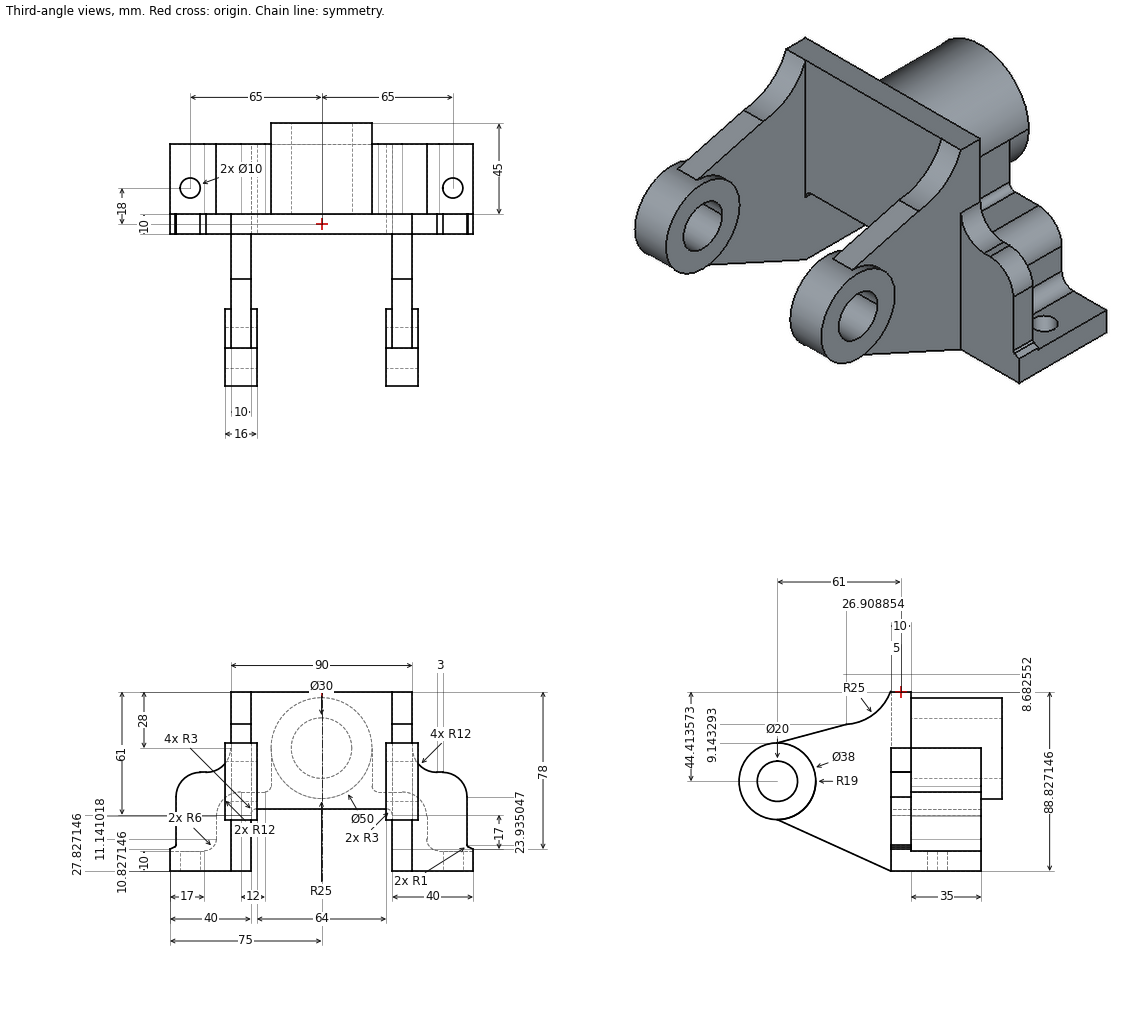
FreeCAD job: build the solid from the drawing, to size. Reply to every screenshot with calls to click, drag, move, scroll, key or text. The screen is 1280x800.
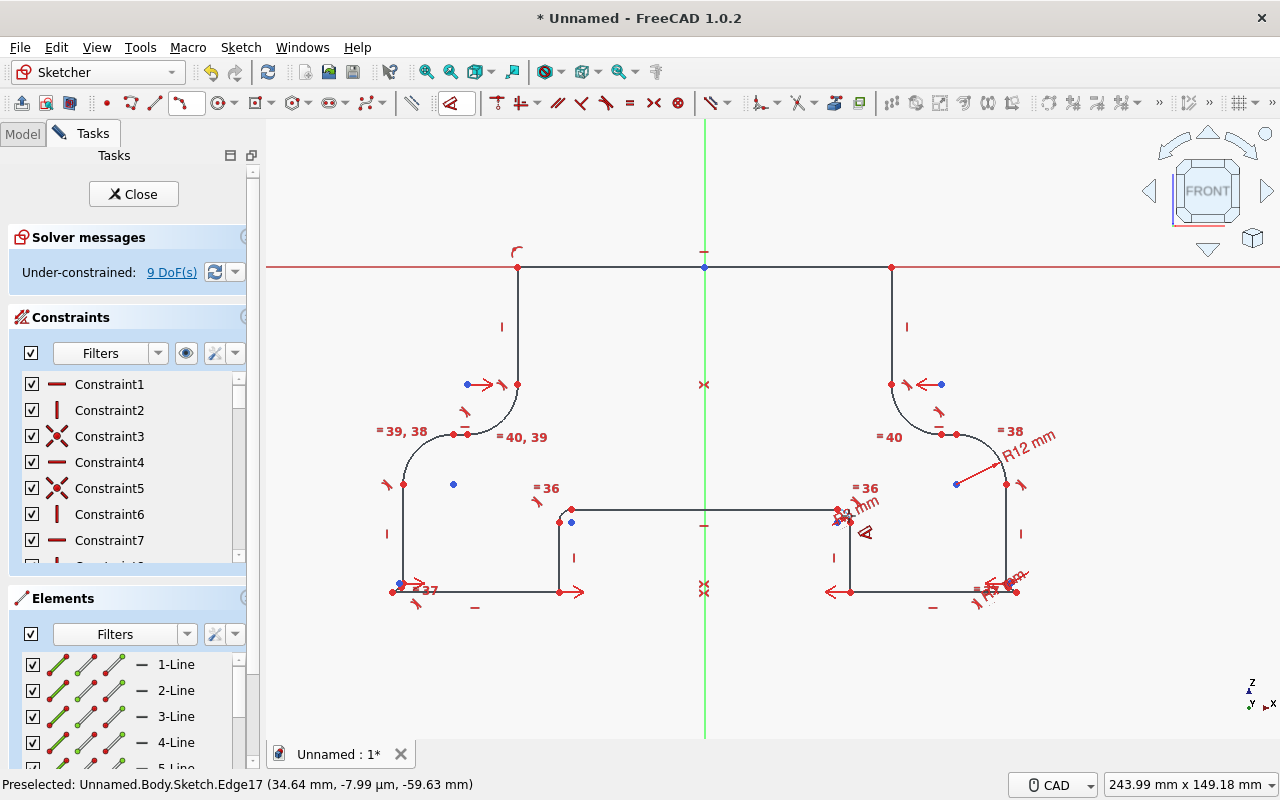
scroll(946, 435, up, 6)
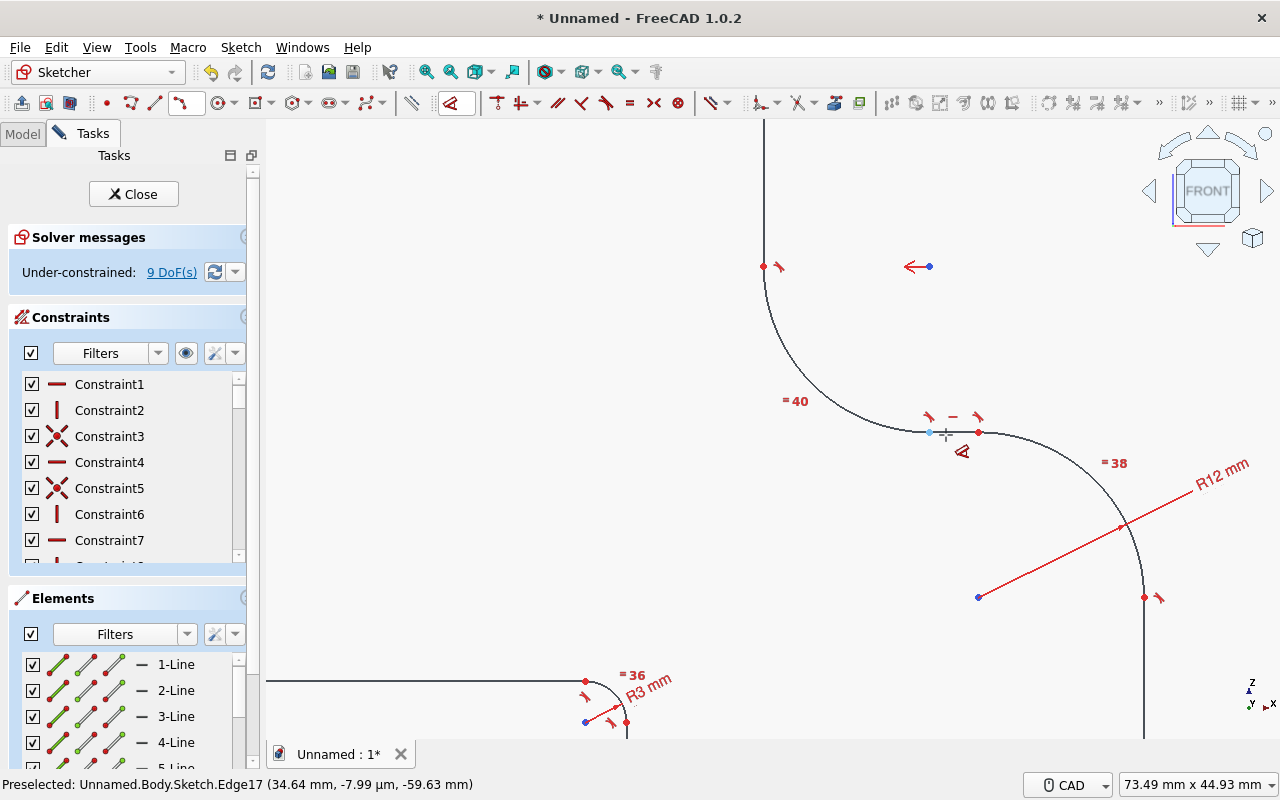
click(944, 432)
click(954, 466)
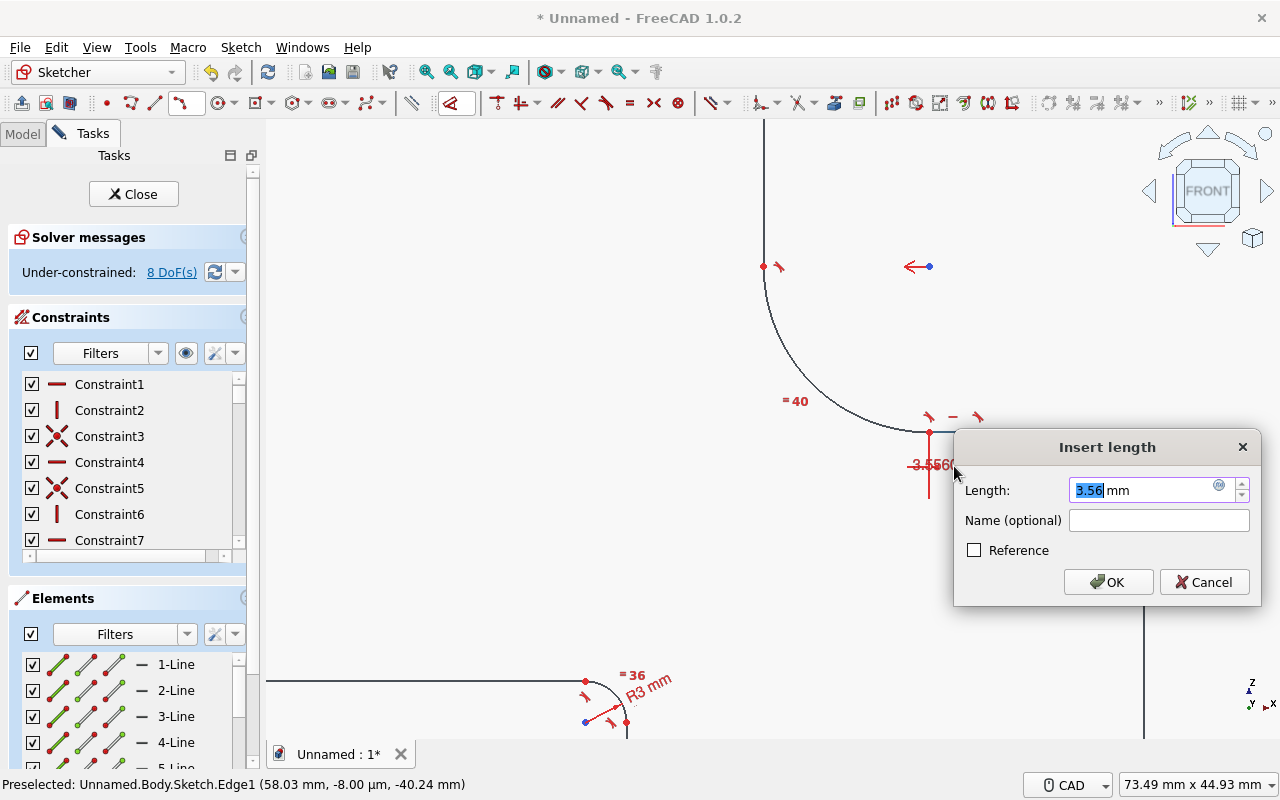
text(3)
key(Return)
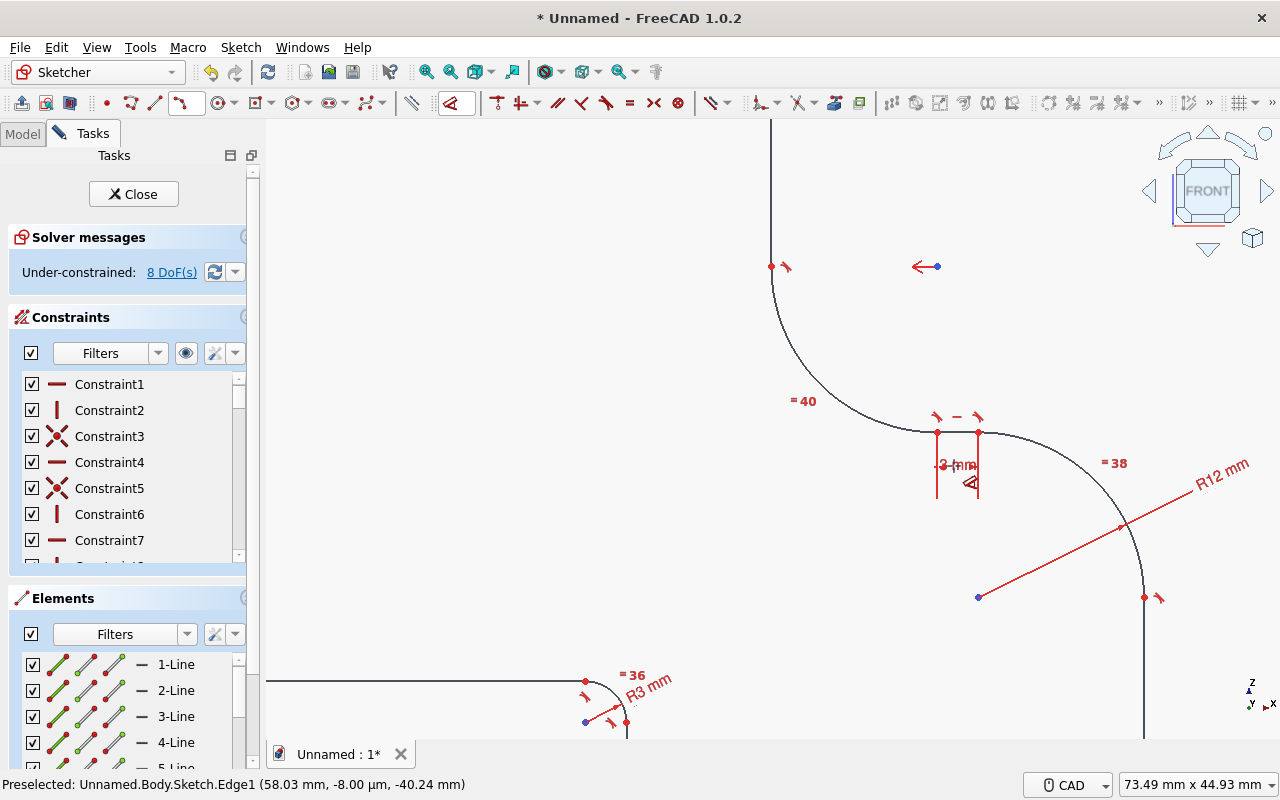
scroll(946, 435, down, 6)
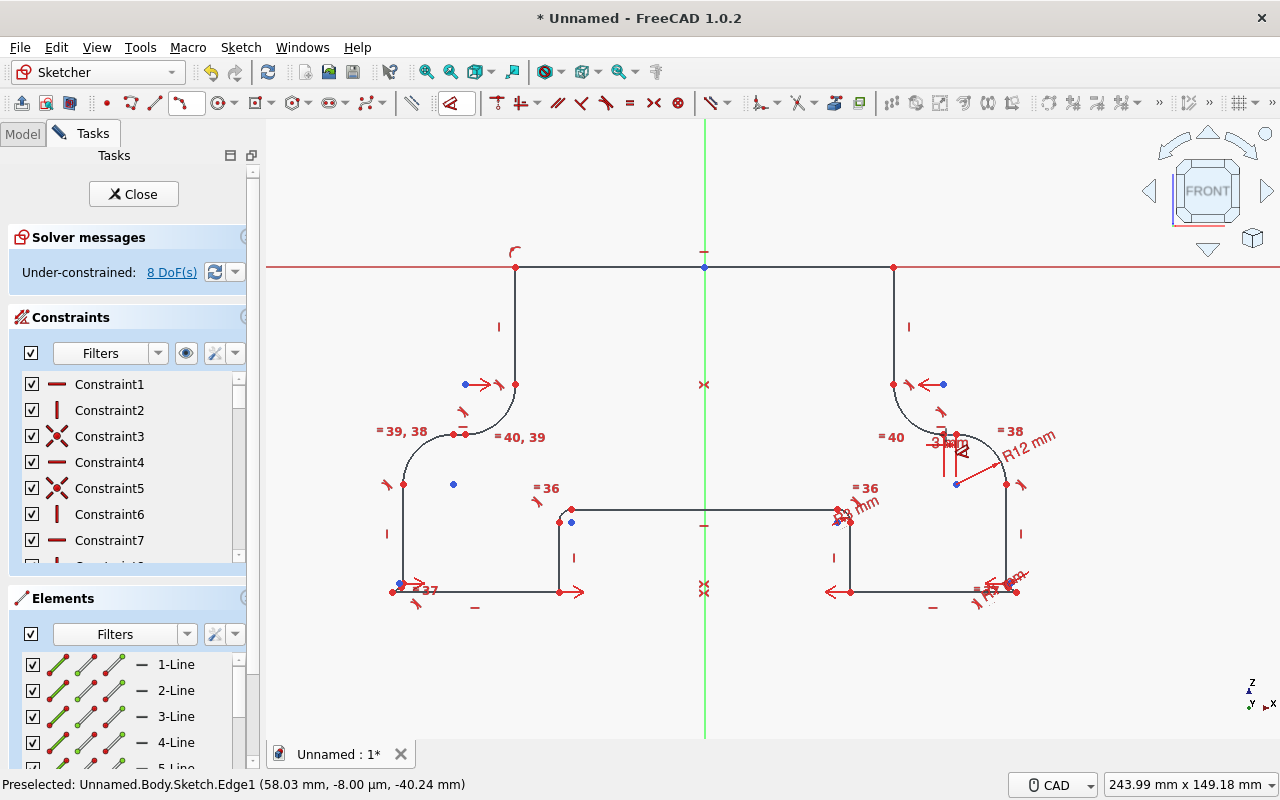
click(967, 592)
click(933, 626)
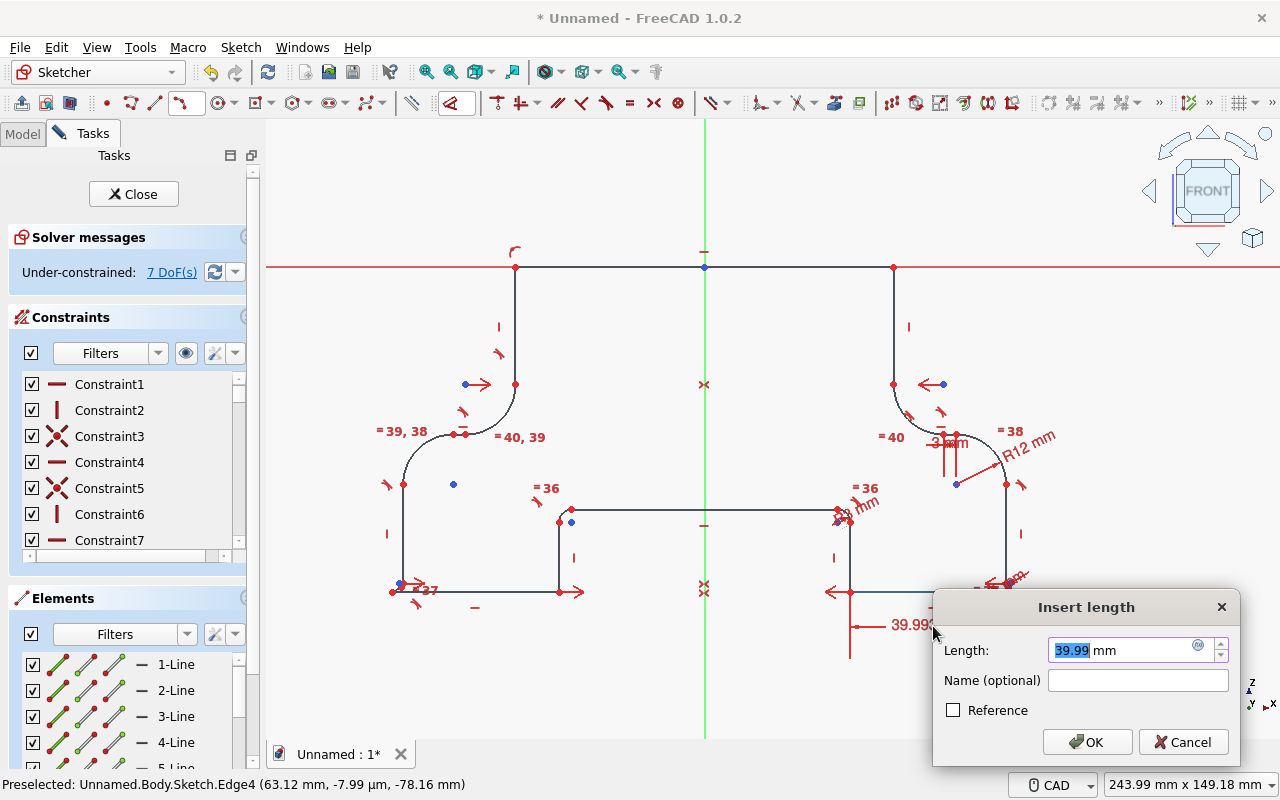
text(40)
key(Return)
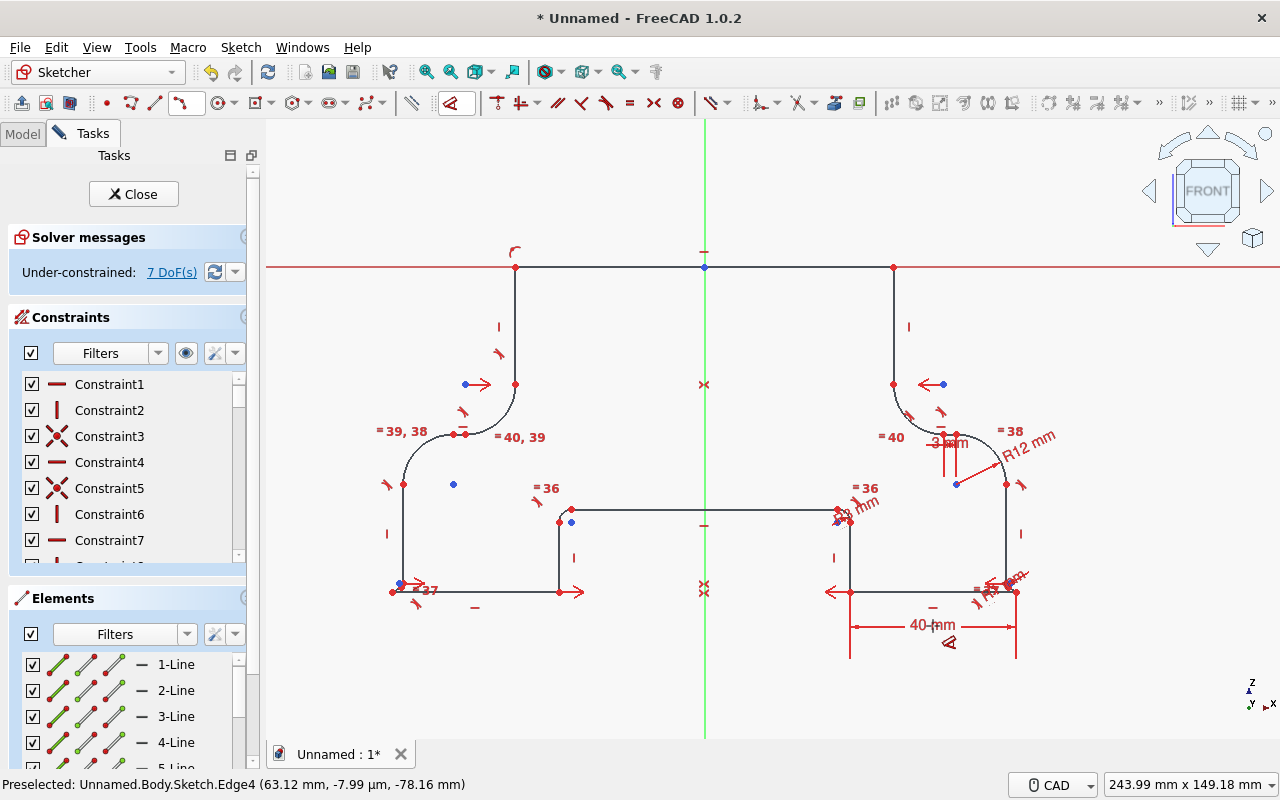
click(850, 571)
click(884, 557)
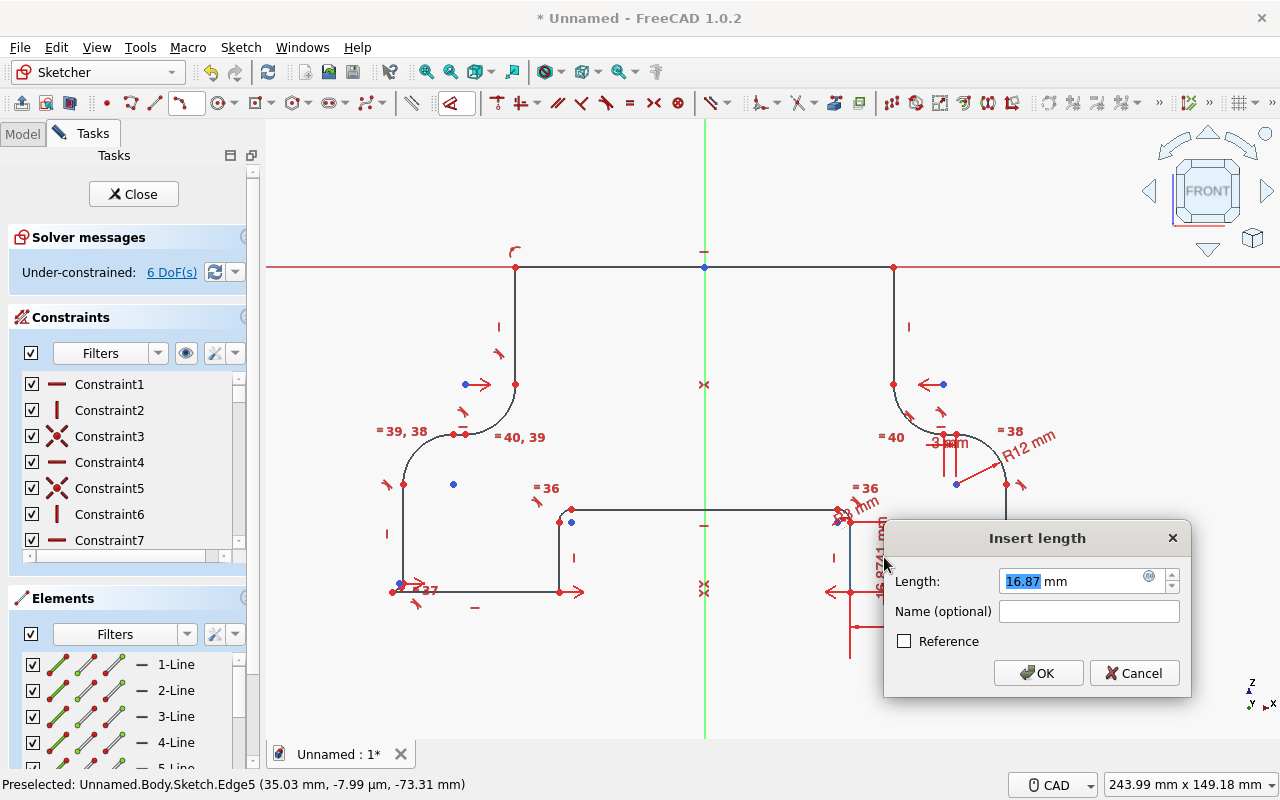
text(17)
key(Return)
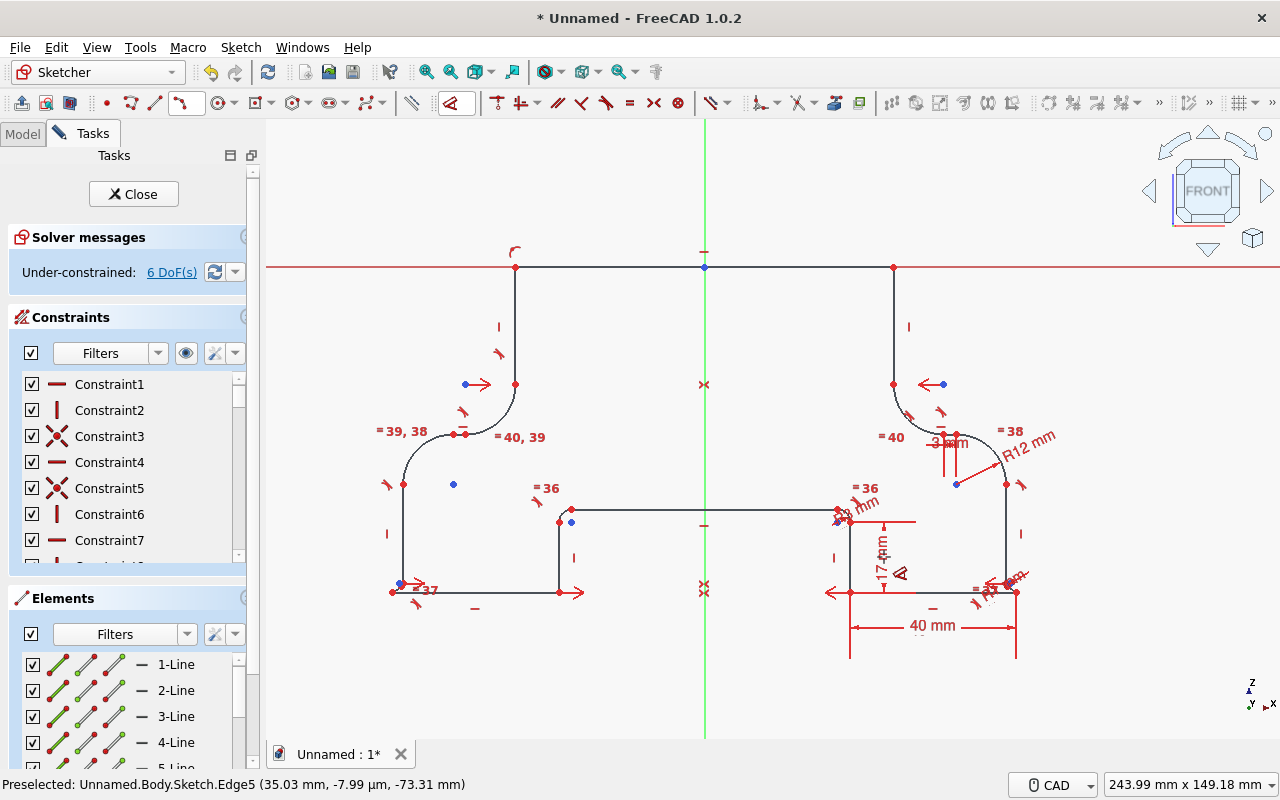
click(758, 510)
click(643, 544)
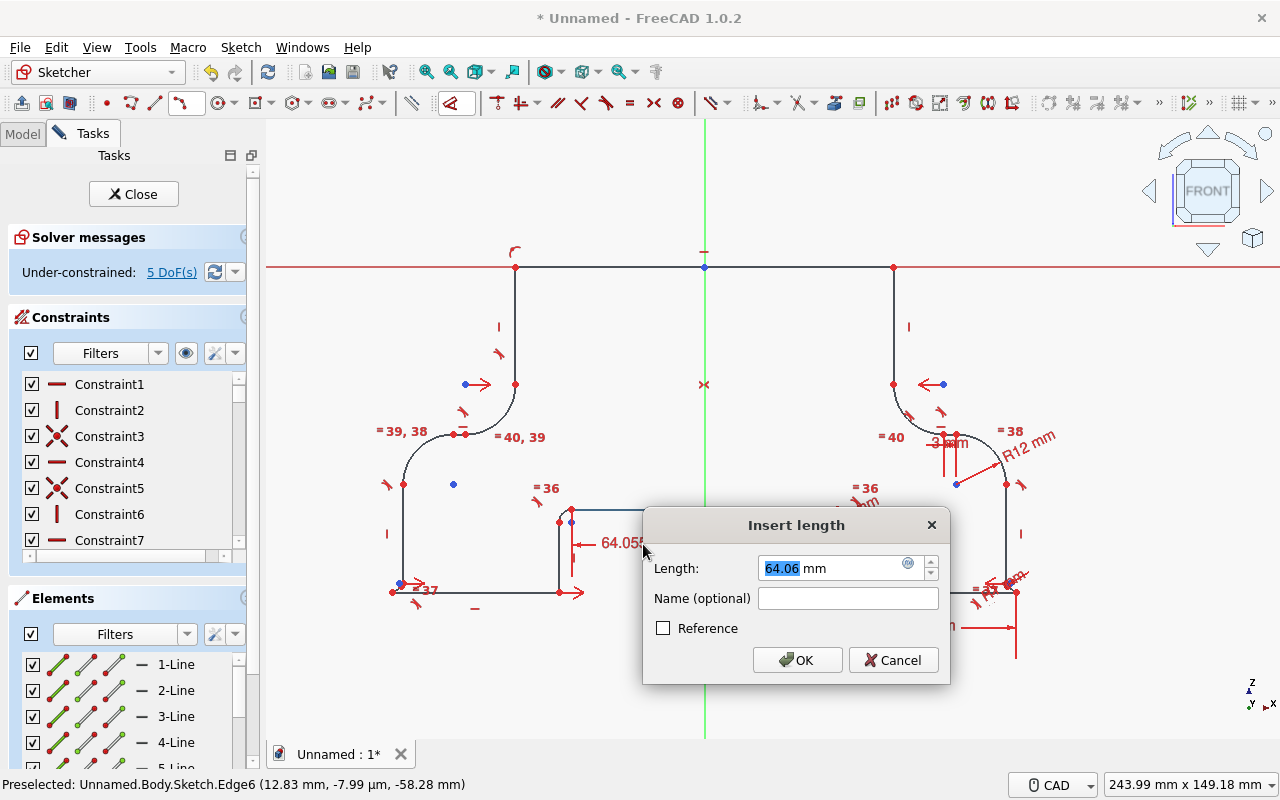
text(64)
key(Return)